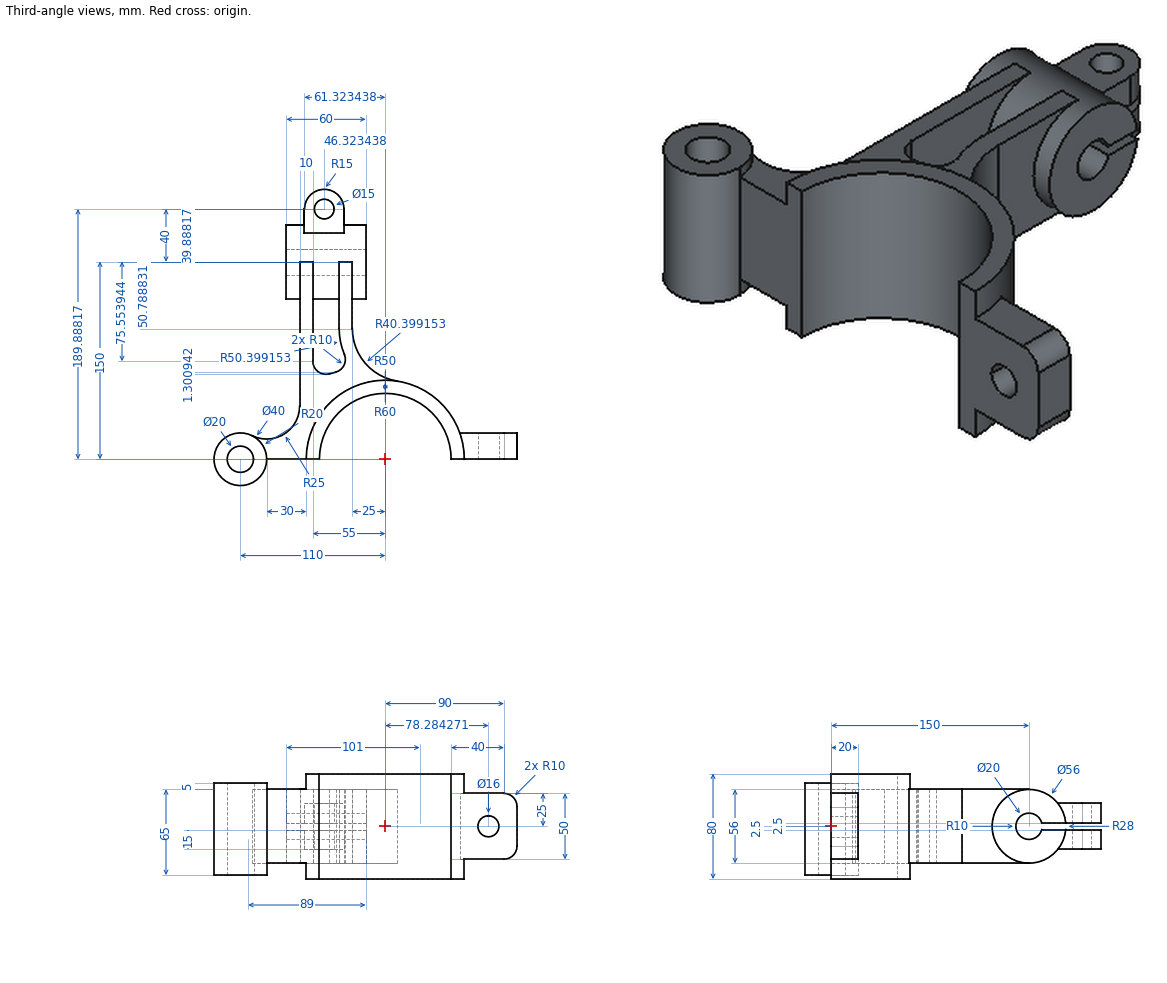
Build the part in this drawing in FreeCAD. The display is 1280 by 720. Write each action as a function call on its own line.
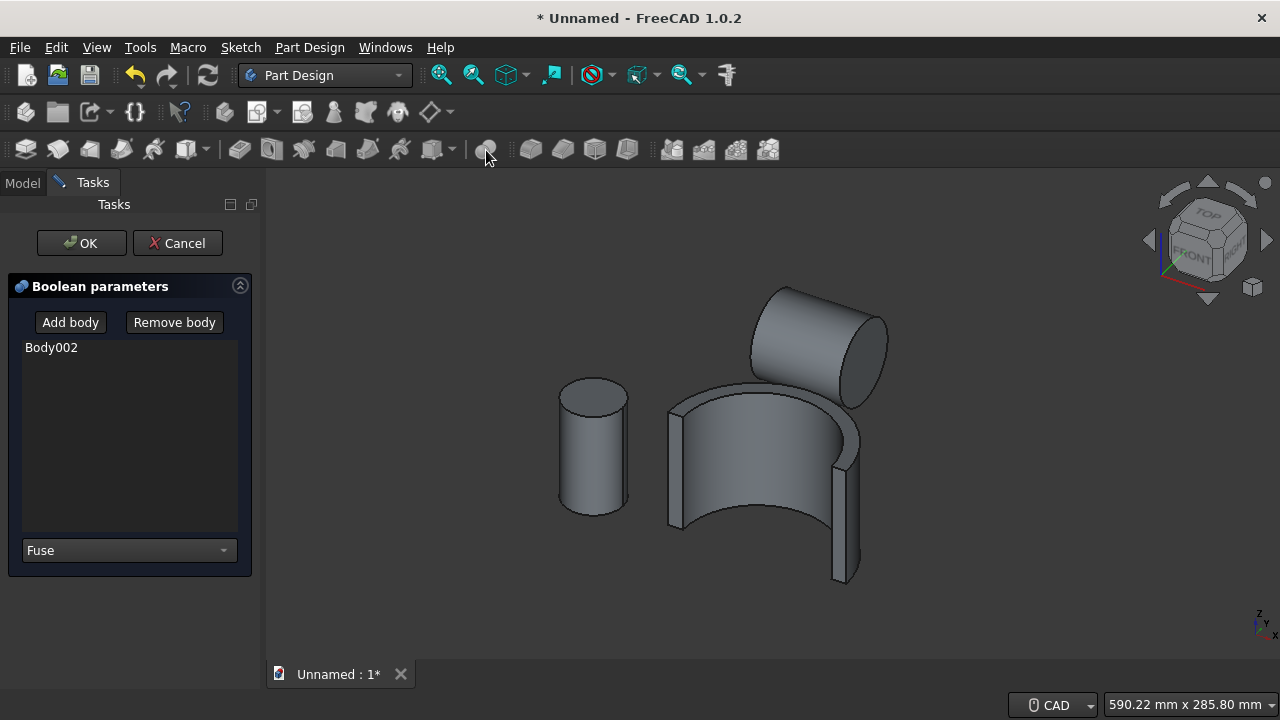
click(82, 243)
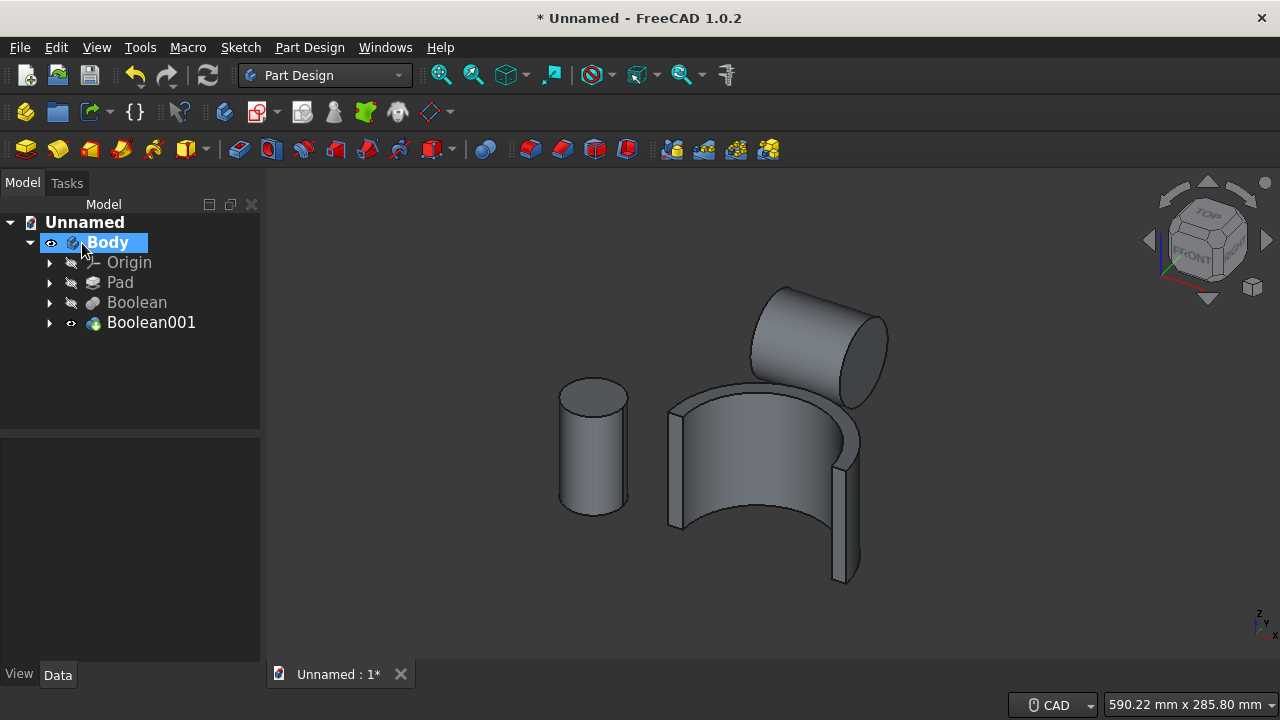
click(258, 112)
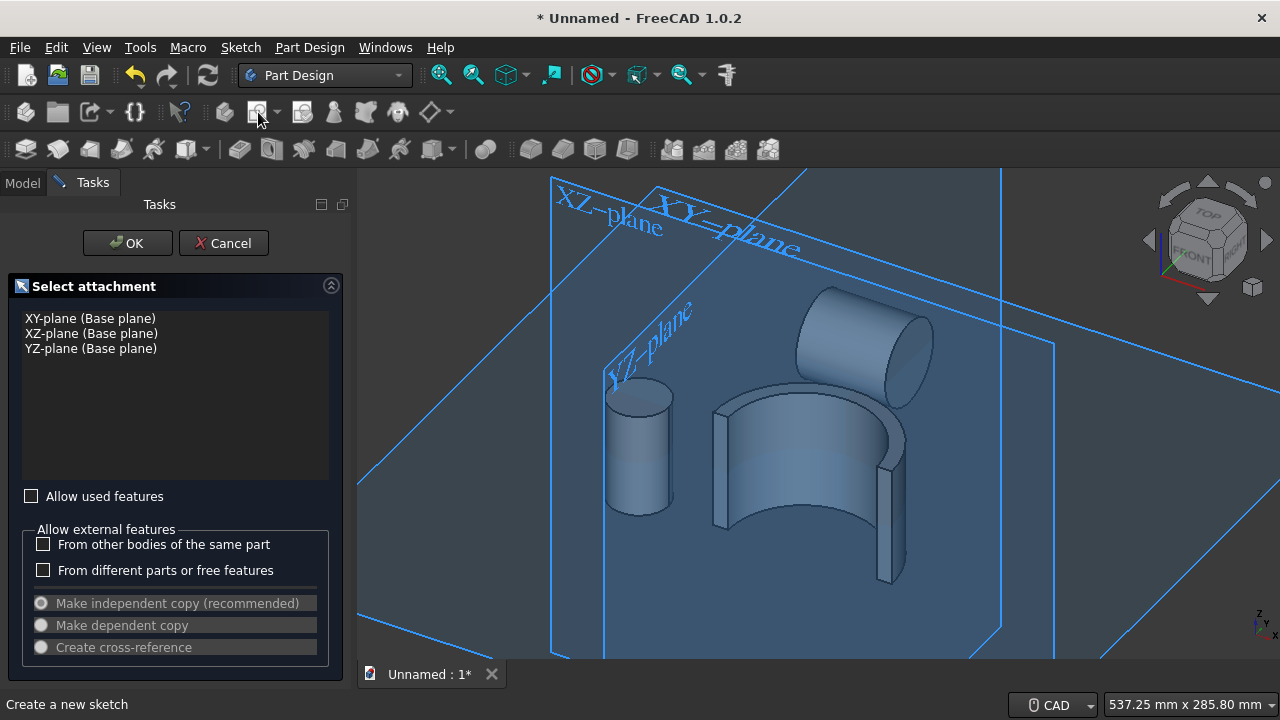
click(82, 318)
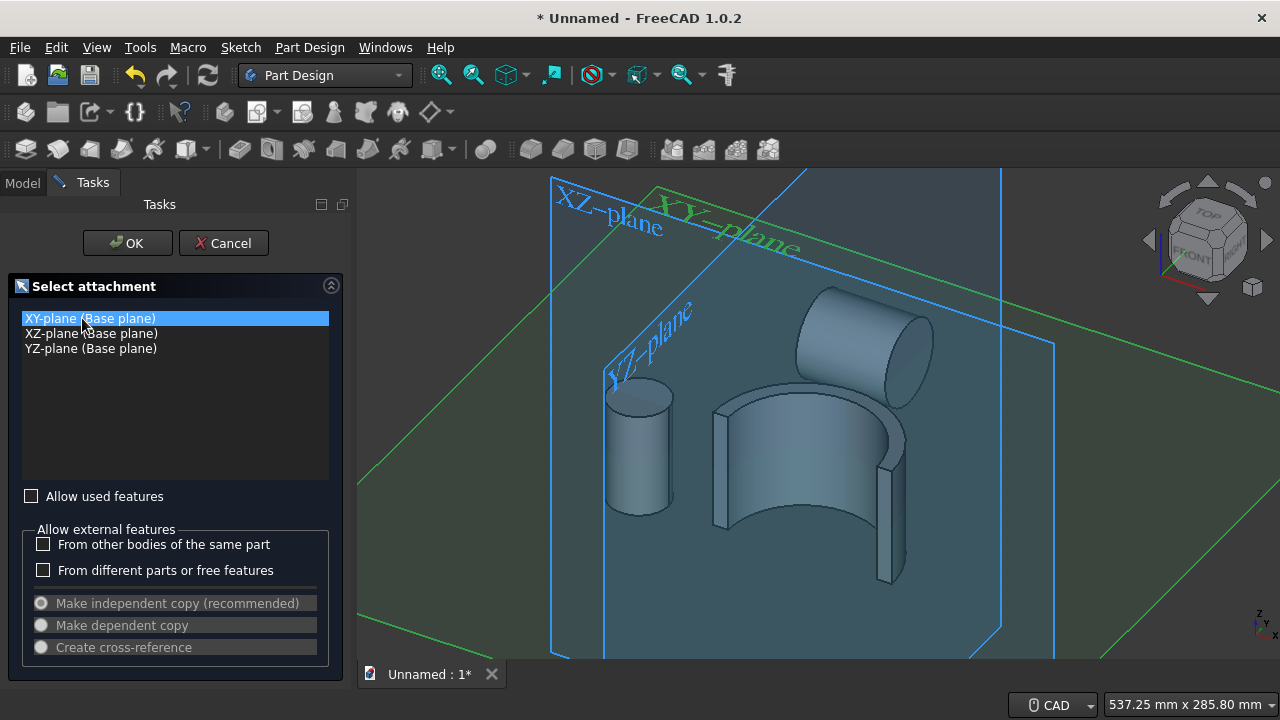
click(128, 243)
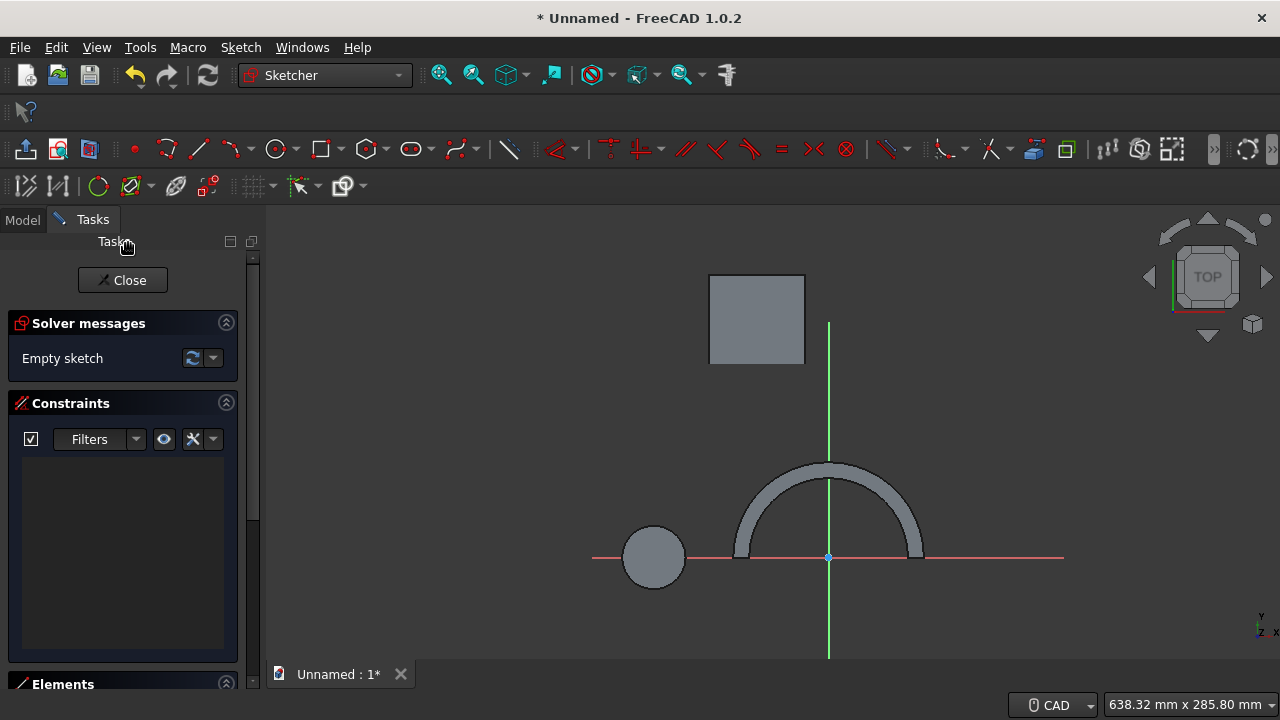
key(q)
key(s)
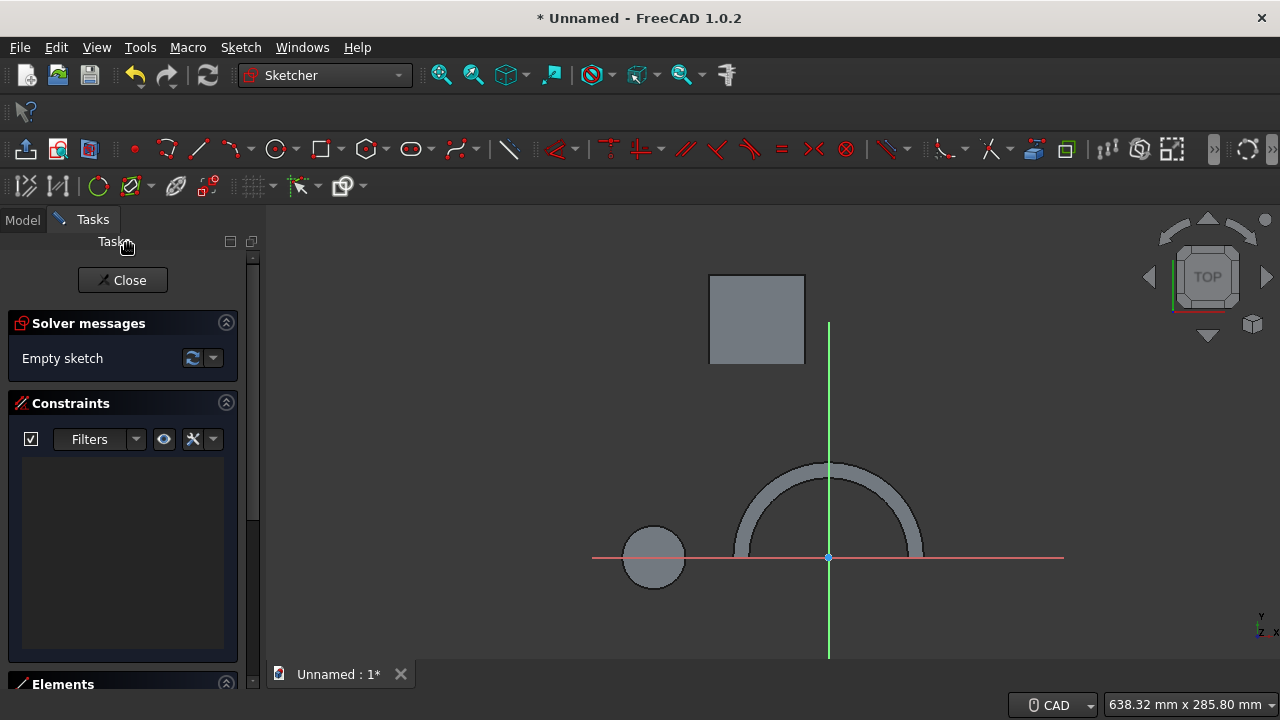
key(g)
key(m)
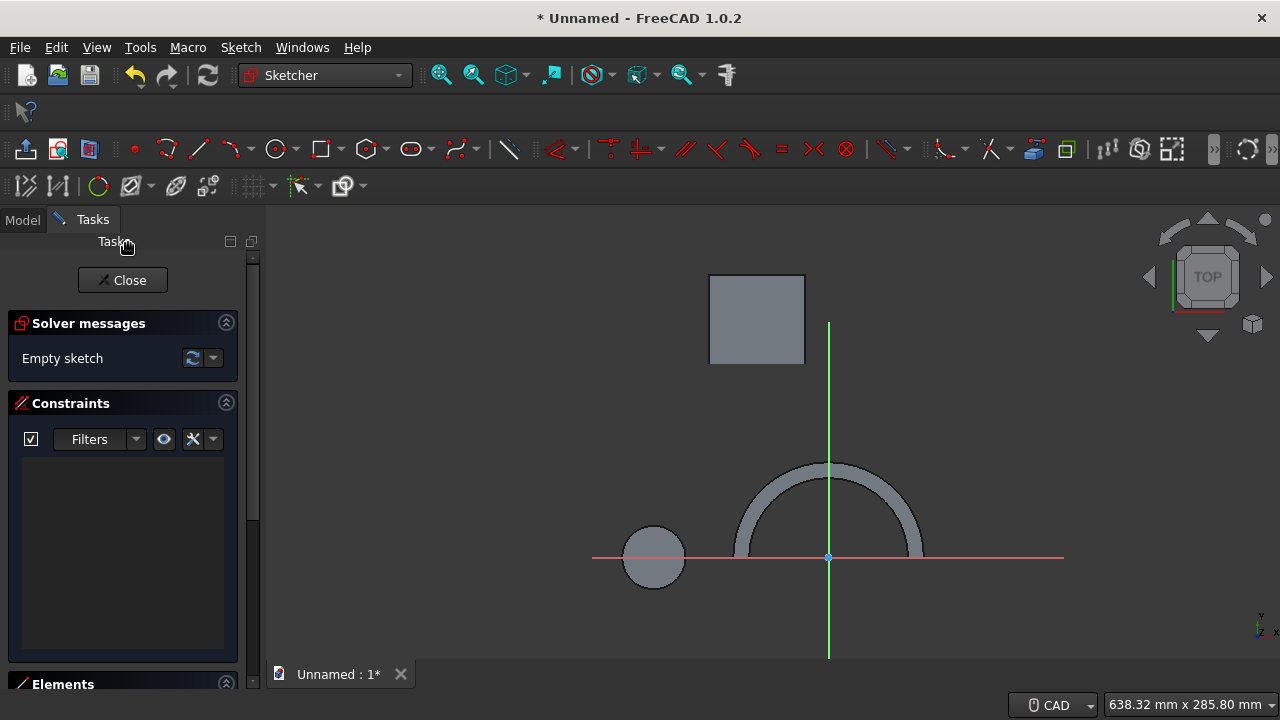
click(741, 439)
click(741, 319)
click(725, 319)
click(725, 493)
right_click(725, 493)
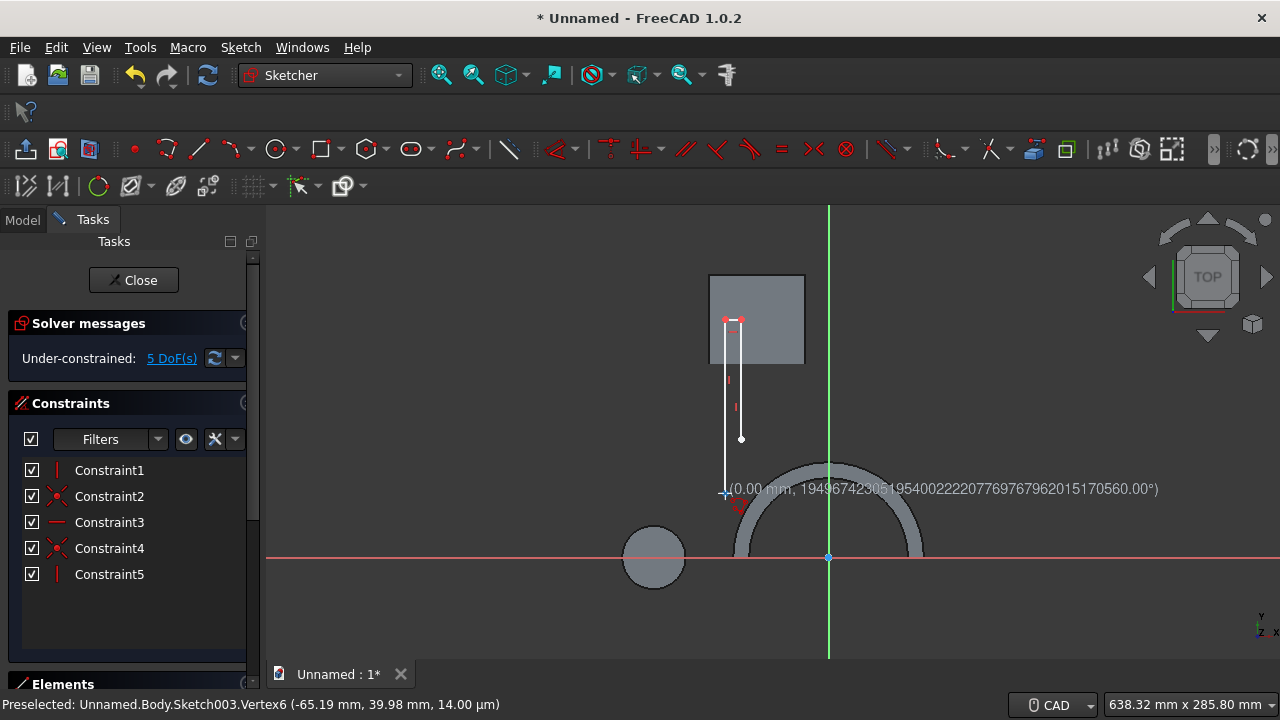
click(200, 150)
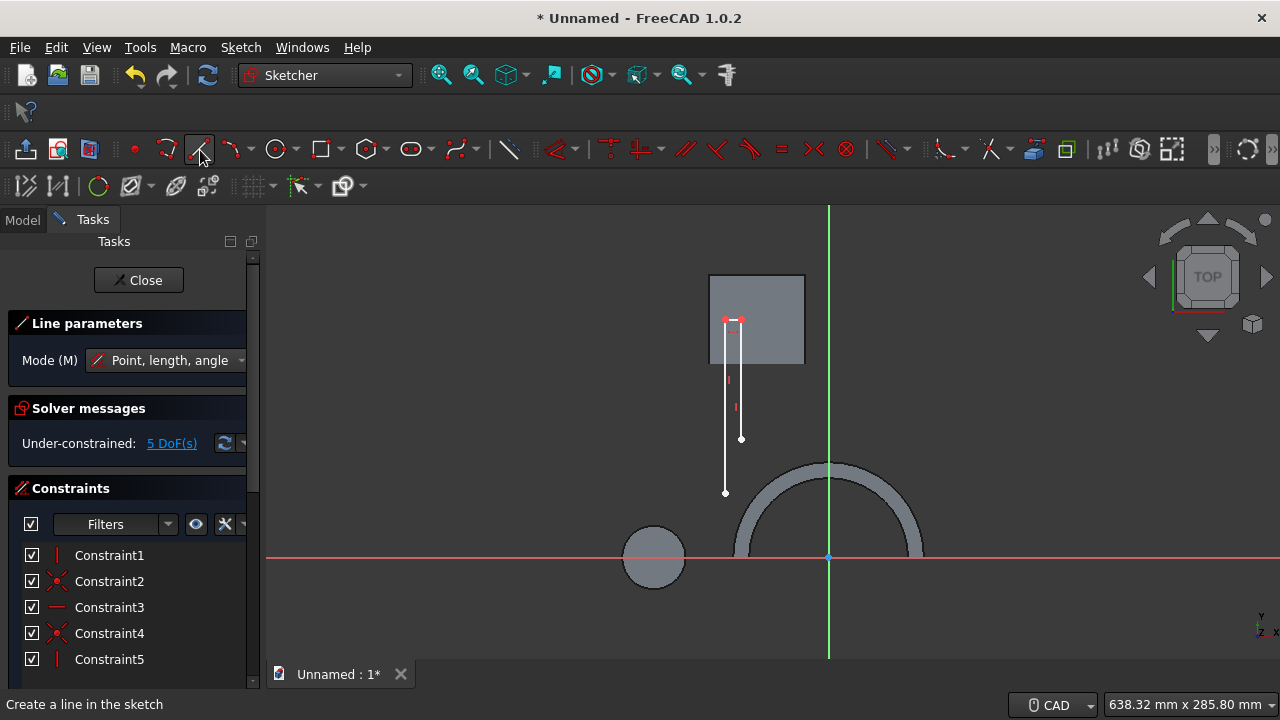
click(686, 558)
click(733, 549)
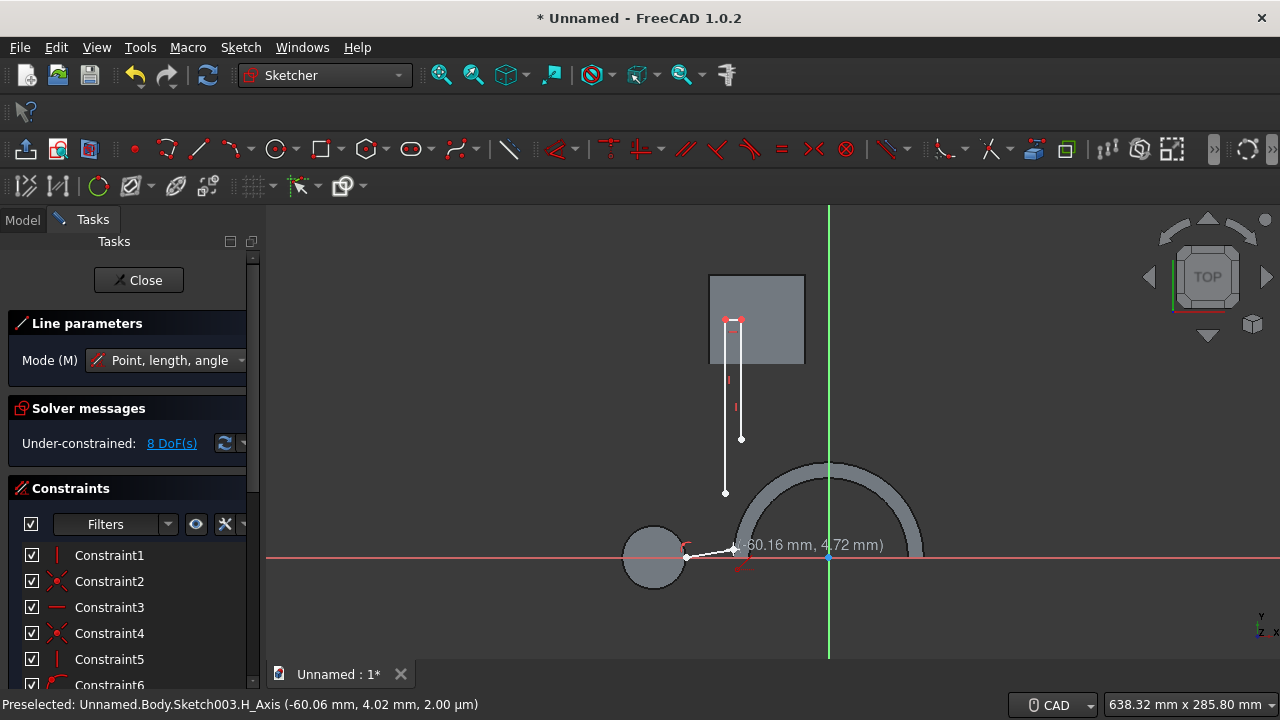
key(g)
key(m)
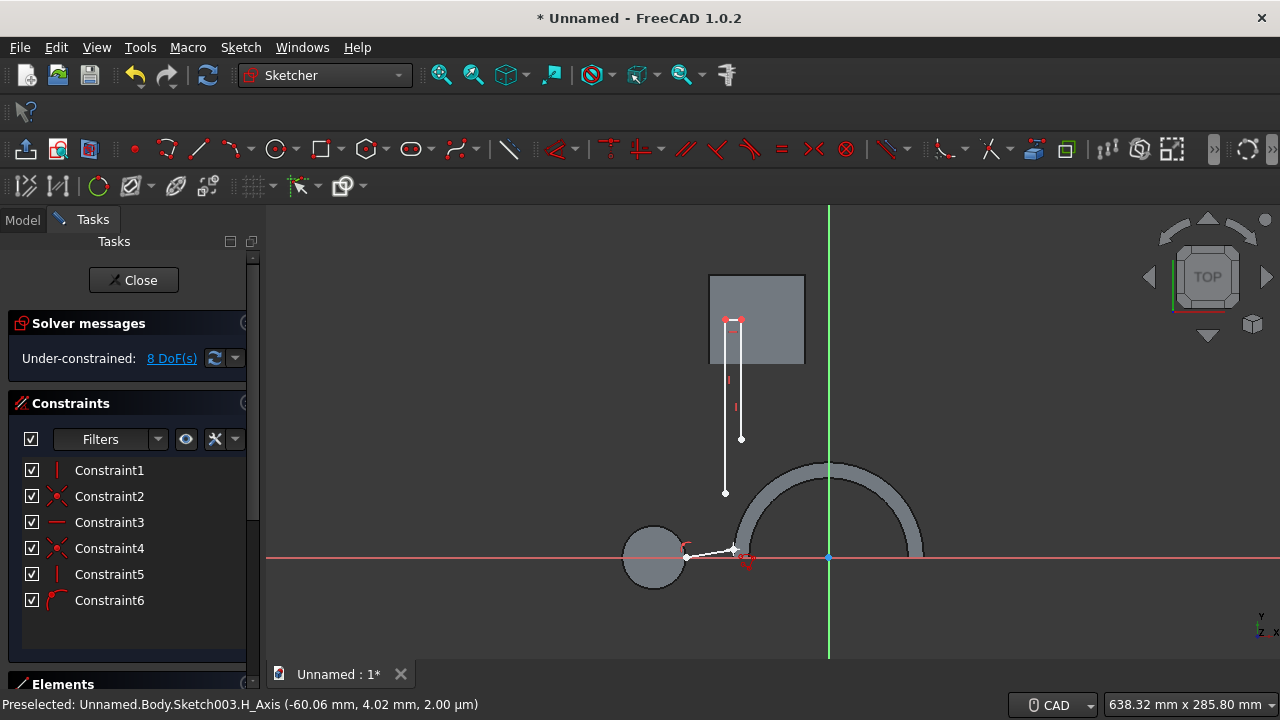
click(789, 400)
click(789, 319)
click(773, 319)
click(773, 400)
right_click(773, 400)